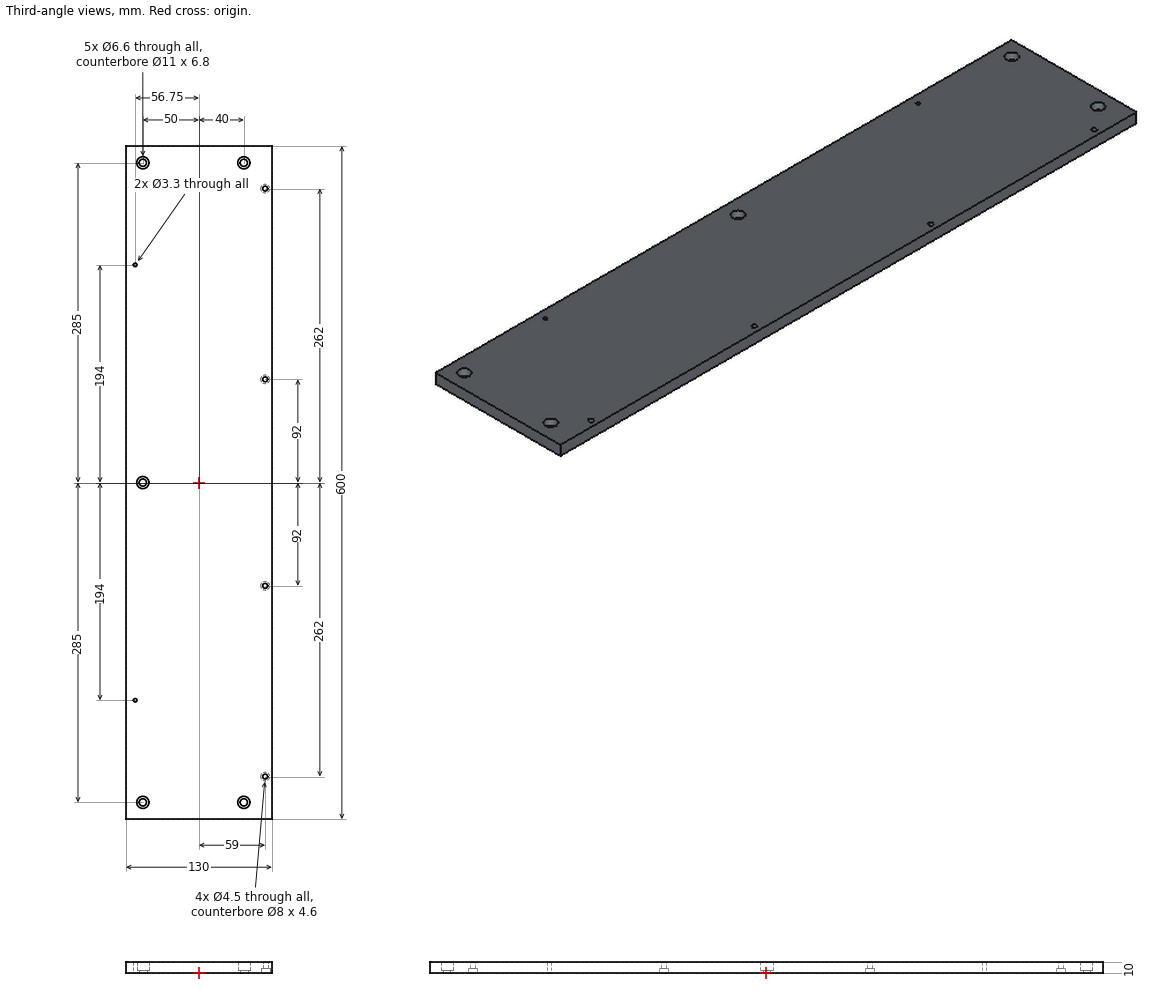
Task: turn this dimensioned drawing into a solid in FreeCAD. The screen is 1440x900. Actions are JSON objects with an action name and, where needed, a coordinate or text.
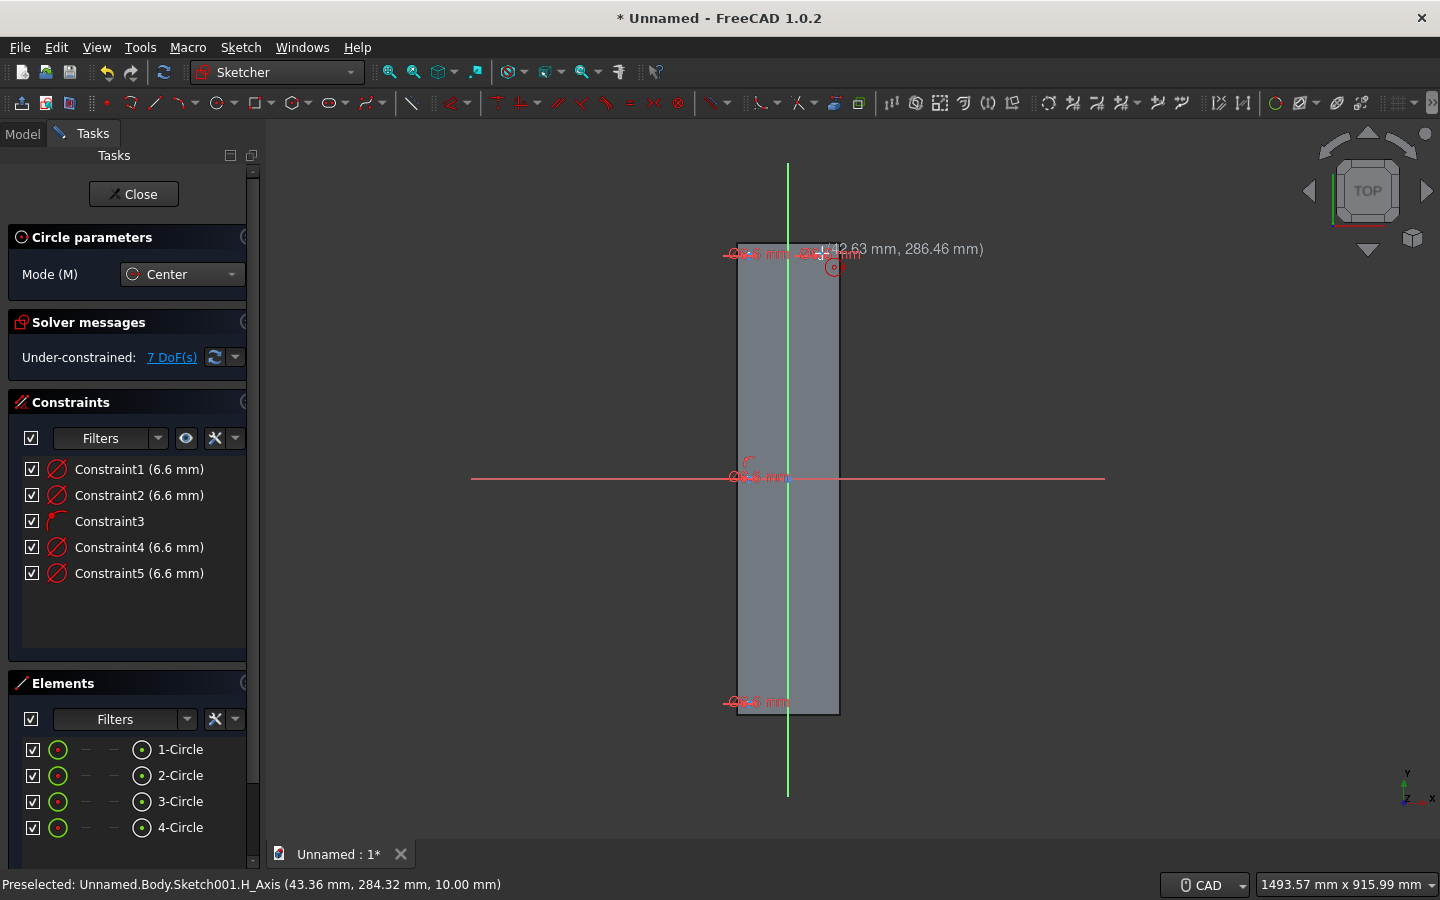
{"action": "scroll", "coordinate": [820, 703], "scroll_direction": "up", "scroll_amount": 11}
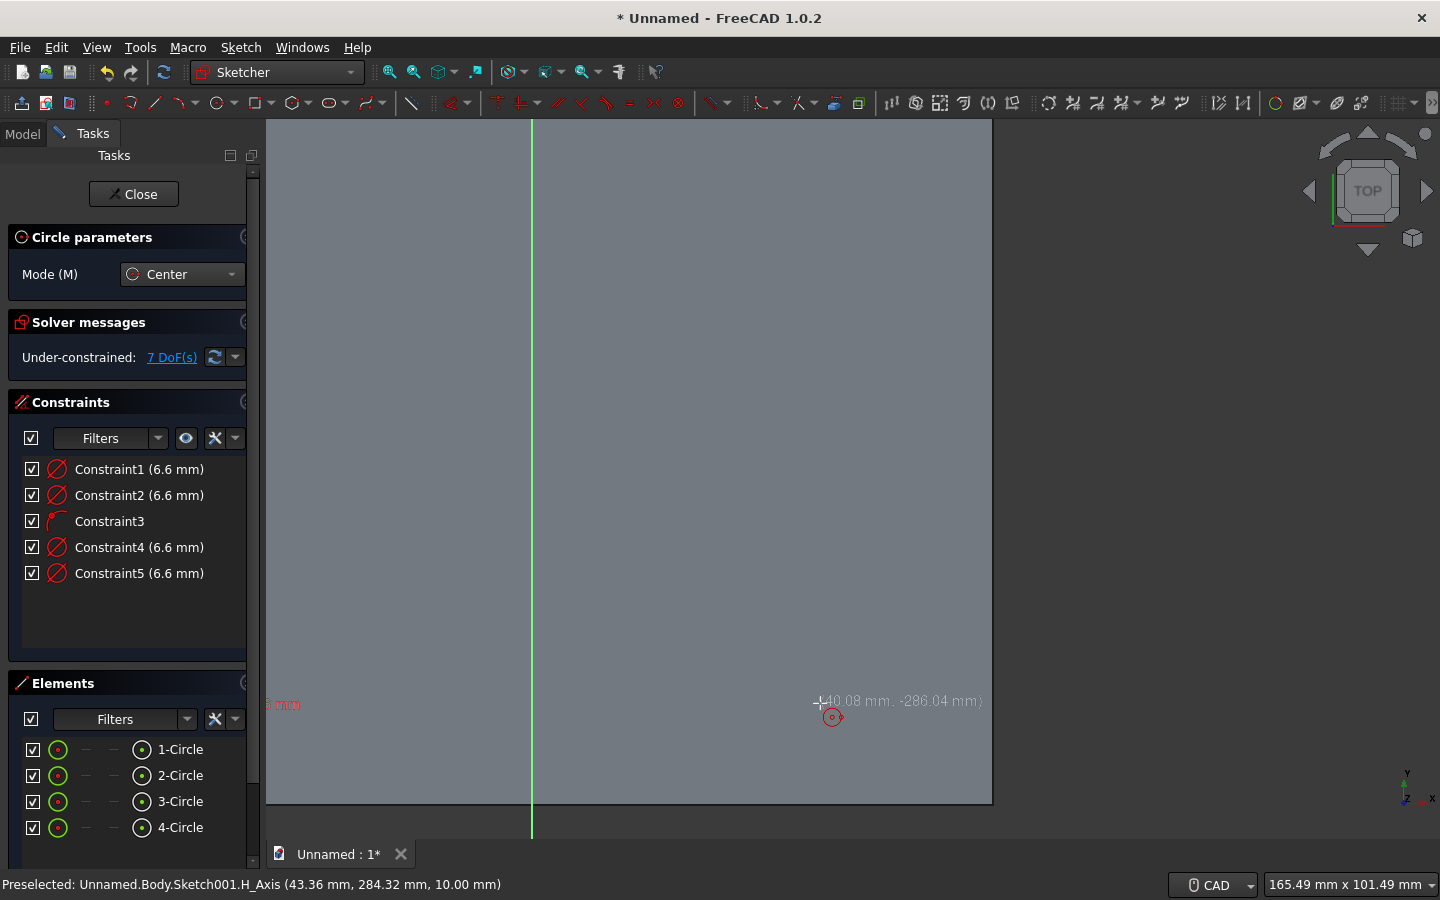
{"action": "scroll", "coordinate": [820, 704], "scroll_direction": "down", "scroll_amount": 11}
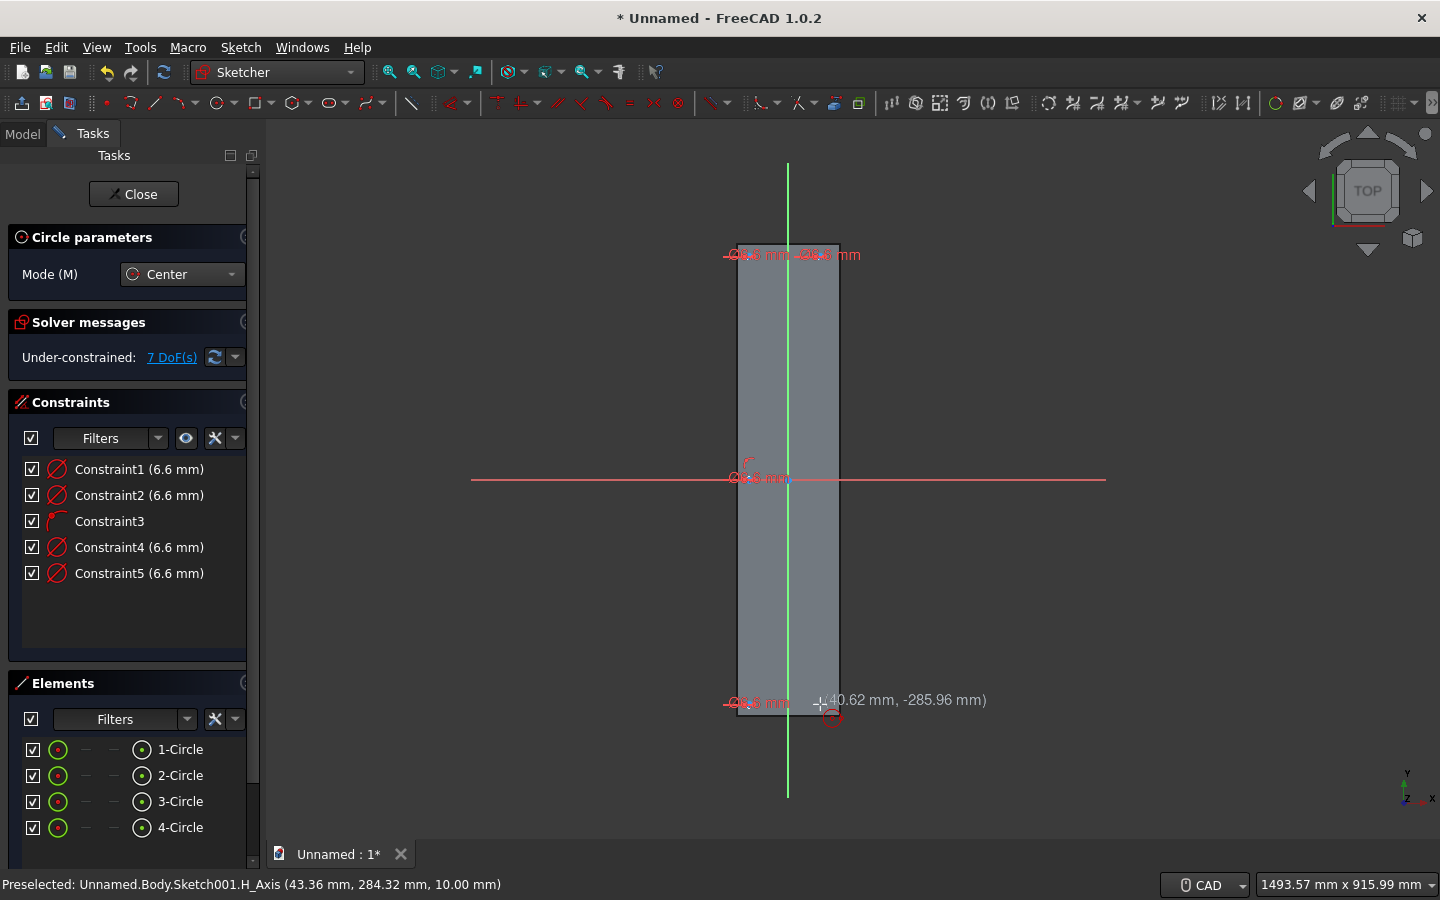
{"action": "left_click", "coordinate": [820, 704]}
{"action": "mouse_move", "coordinate": [822, 702]}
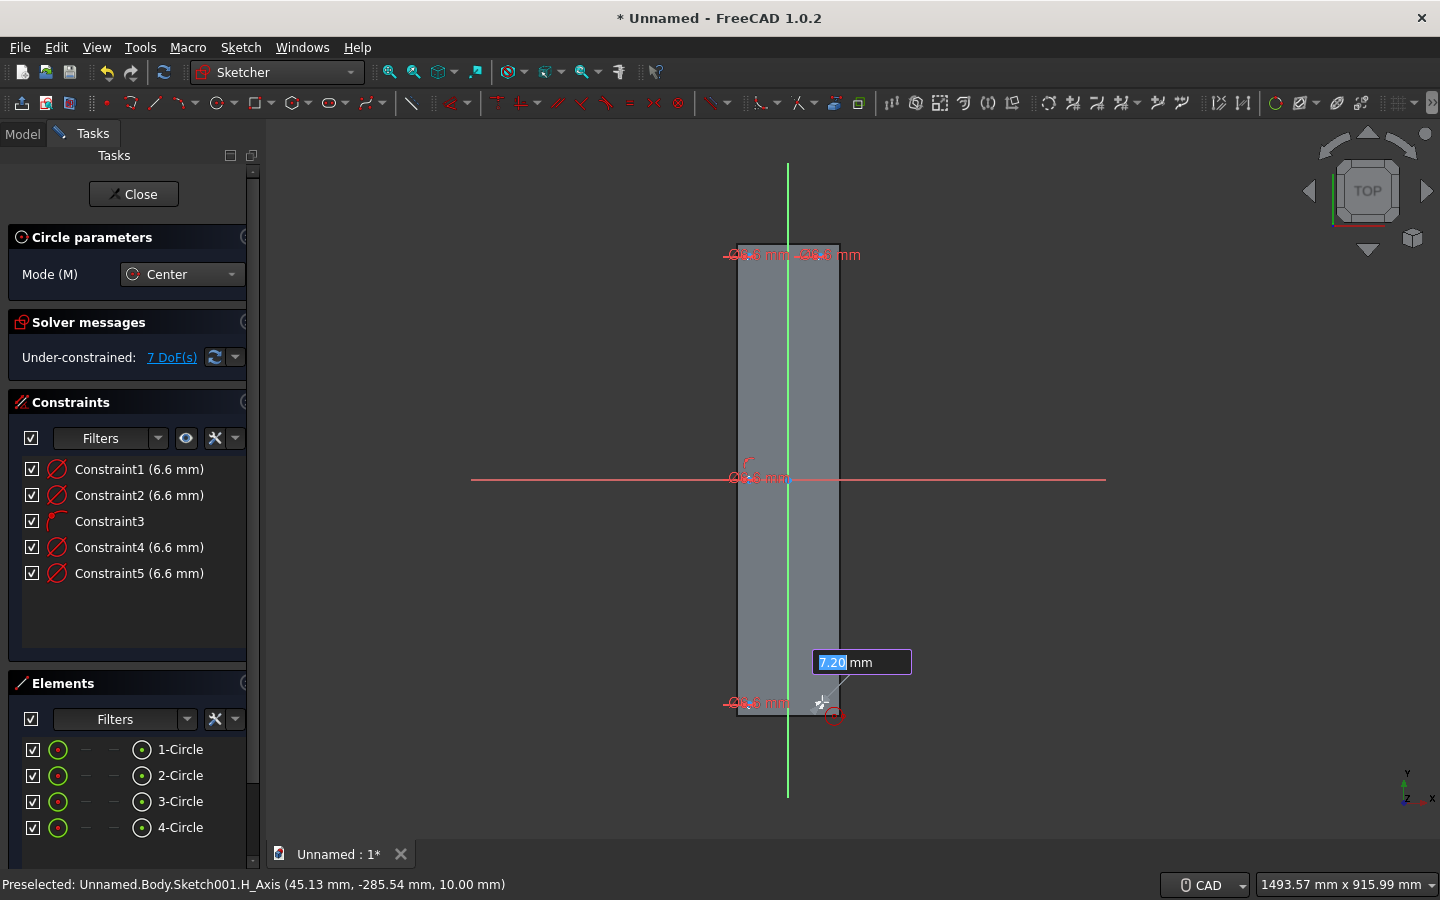
{"action": "type", "text": "6.6"}
{"action": "key", "text": "Return"}
{"action": "key", "text": "Escape"}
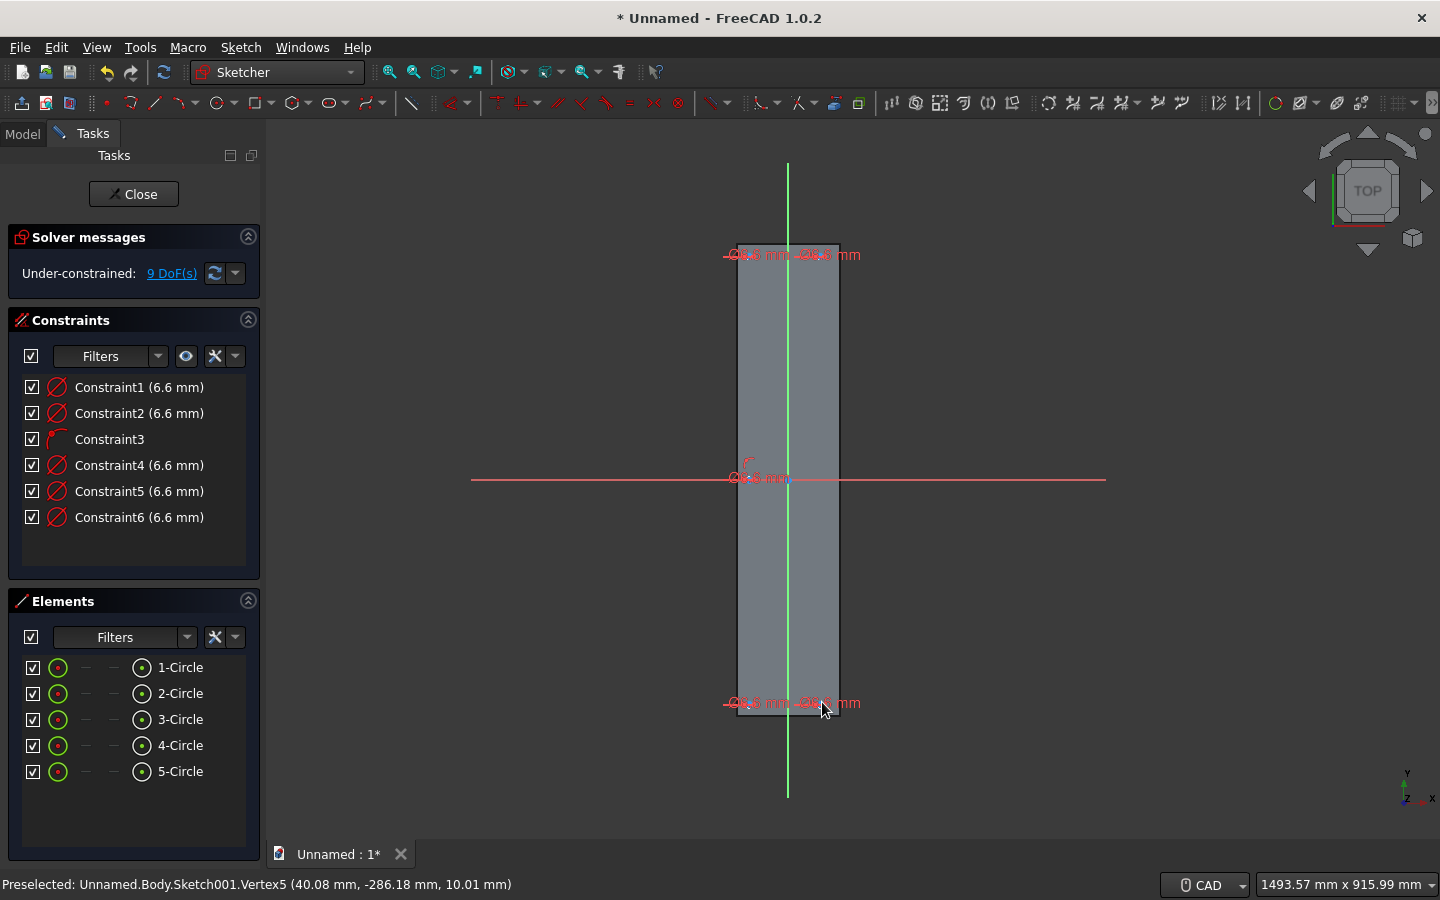
{"action": "left_click", "coordinate": [749, 257]}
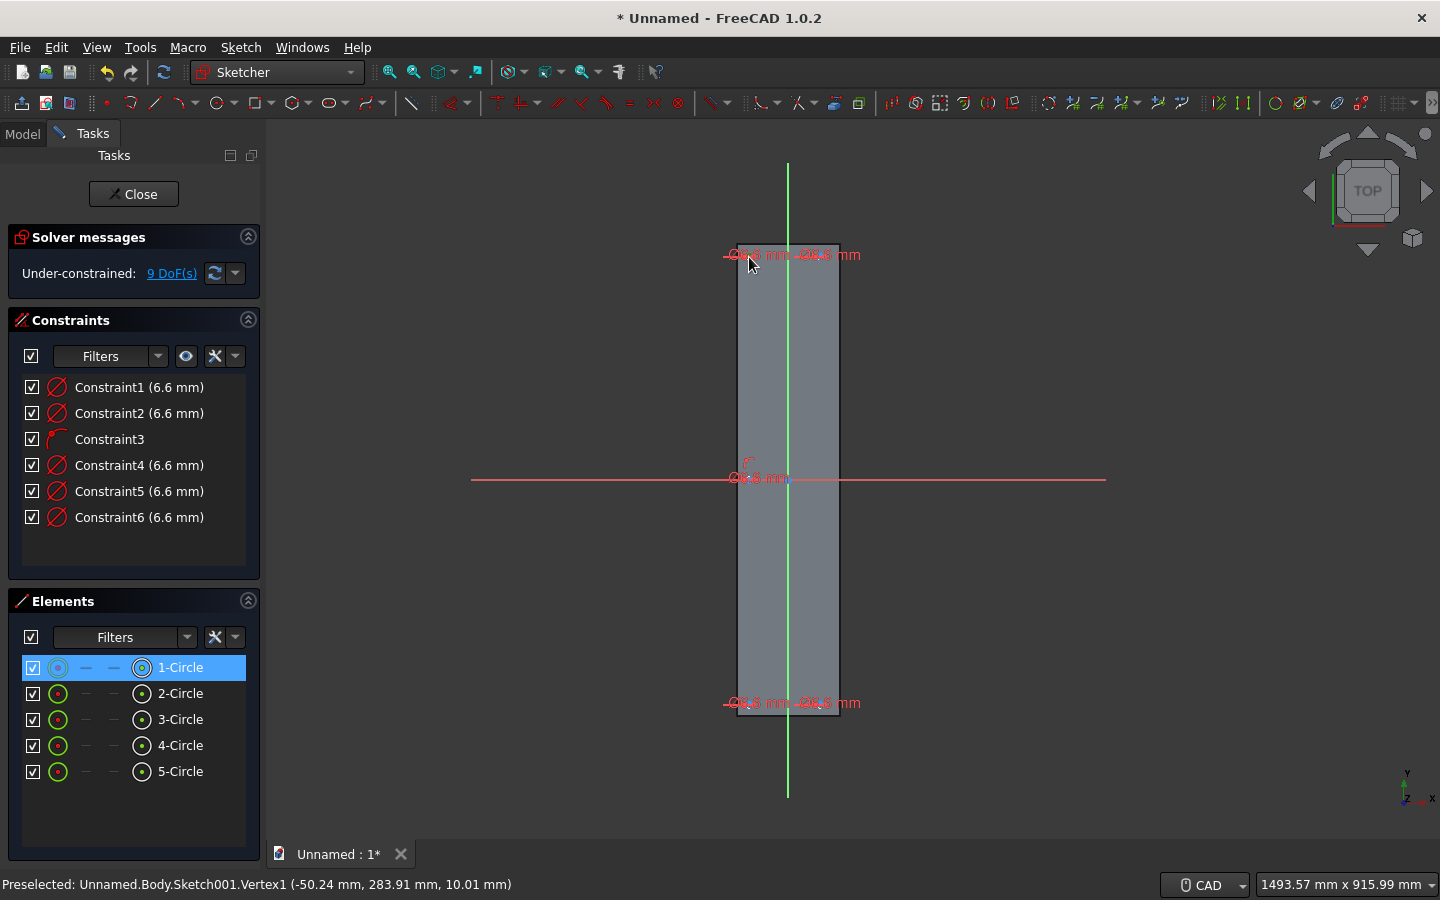
{"action": "left_click", "coordinate": [749, 480]}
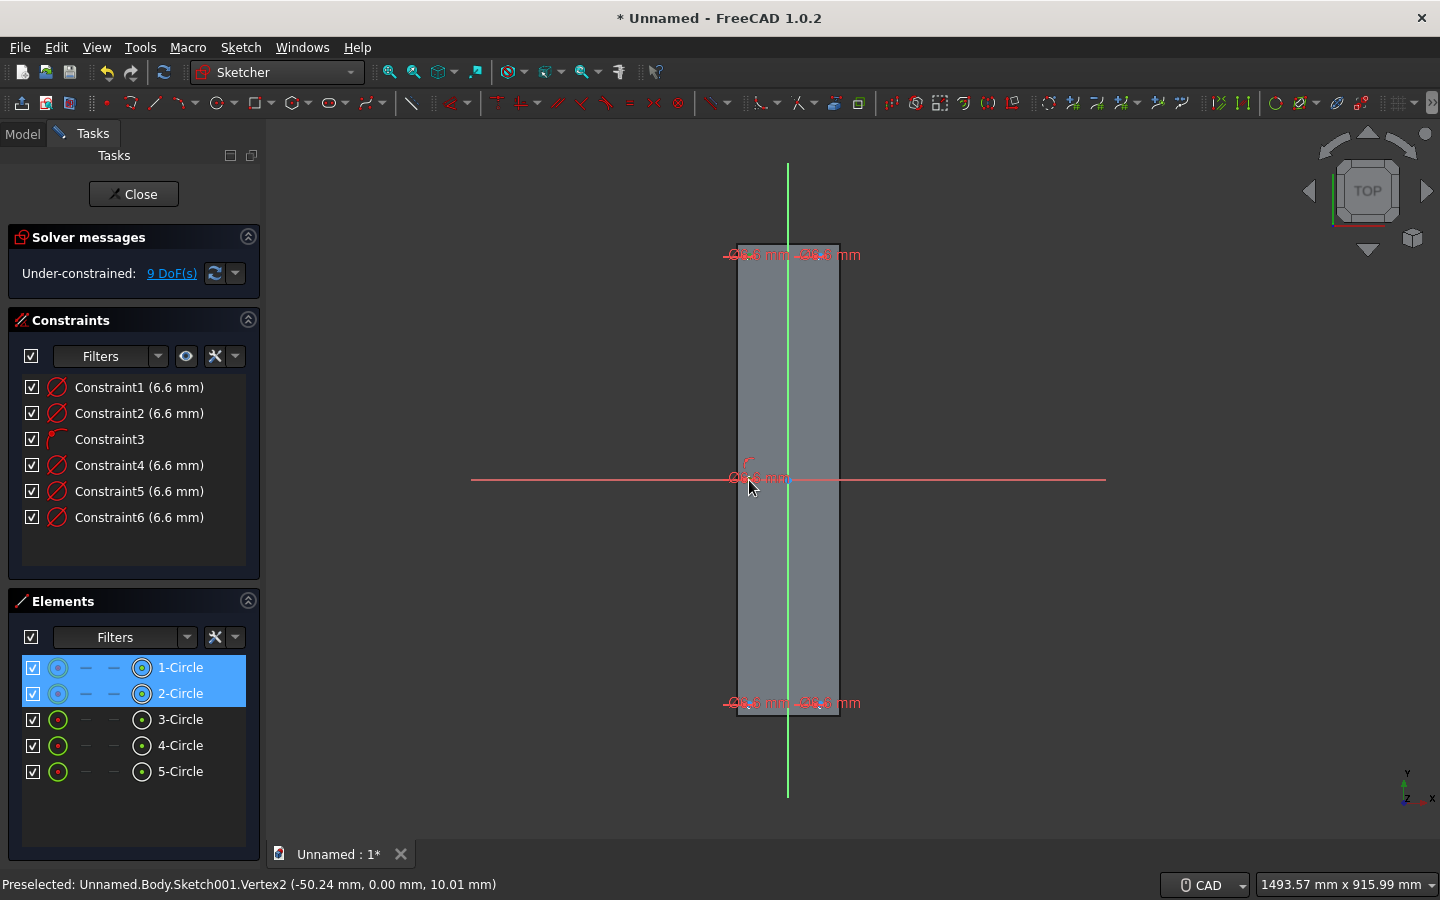
{"action": "key", "text": "v"}